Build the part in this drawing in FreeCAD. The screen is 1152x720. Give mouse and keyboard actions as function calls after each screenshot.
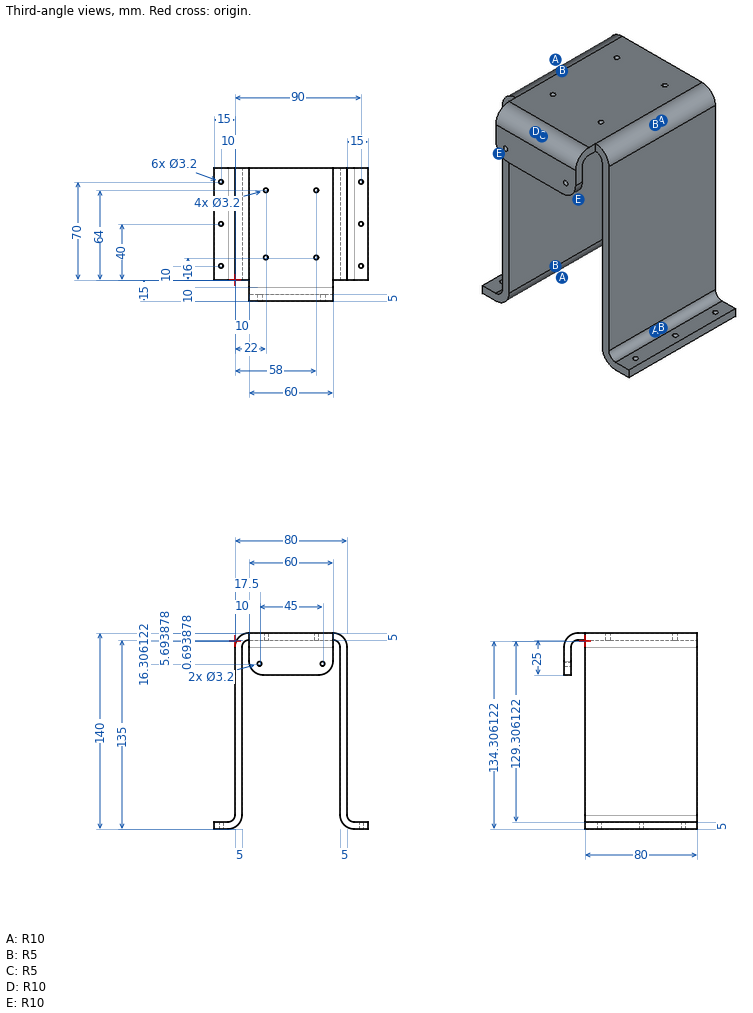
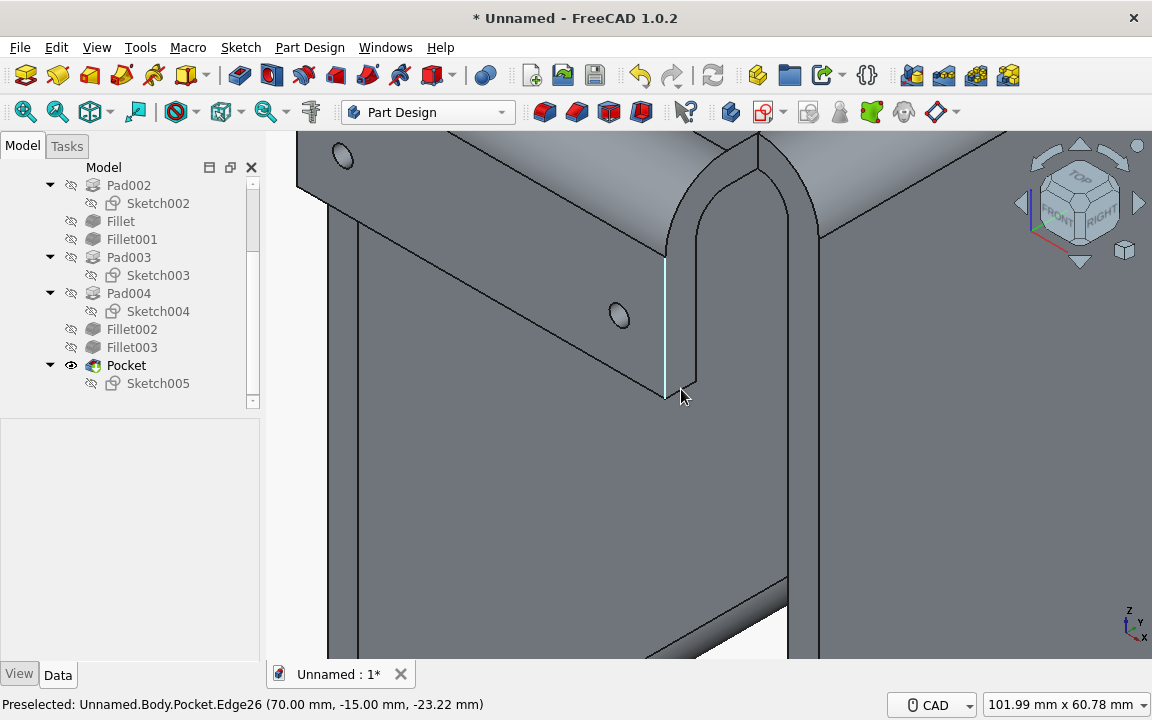
click(26, 112)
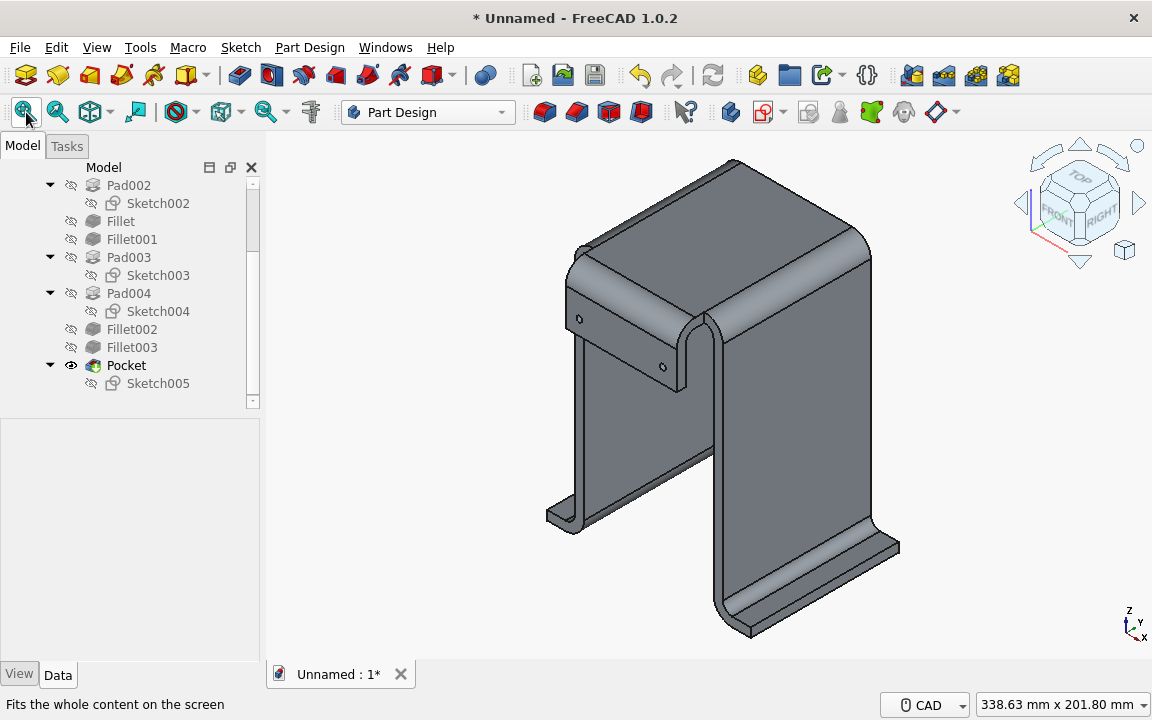
key(2)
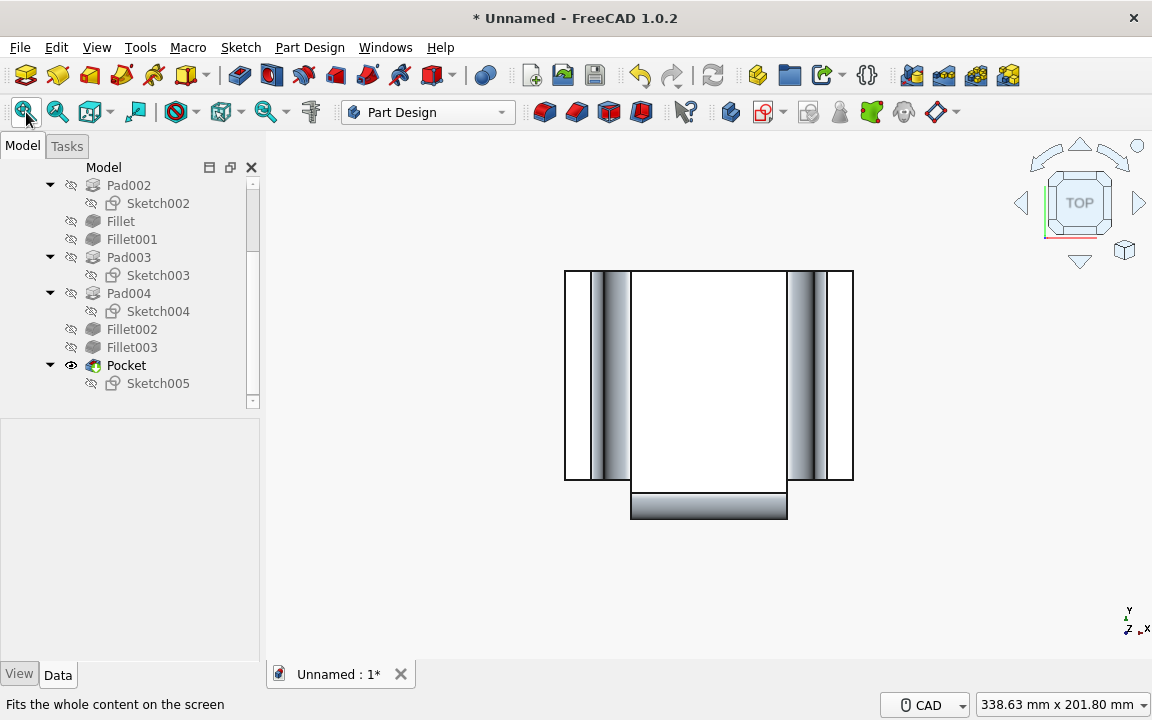
scroll(787, 512, up, 6)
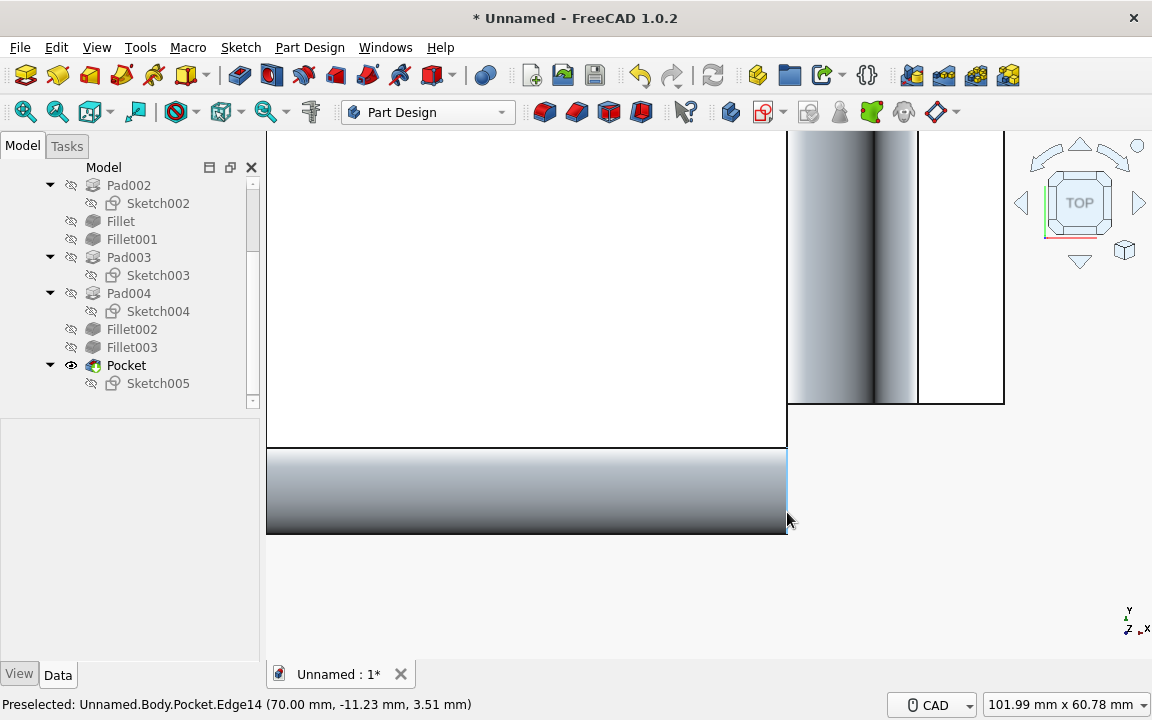
key(v)
key(f)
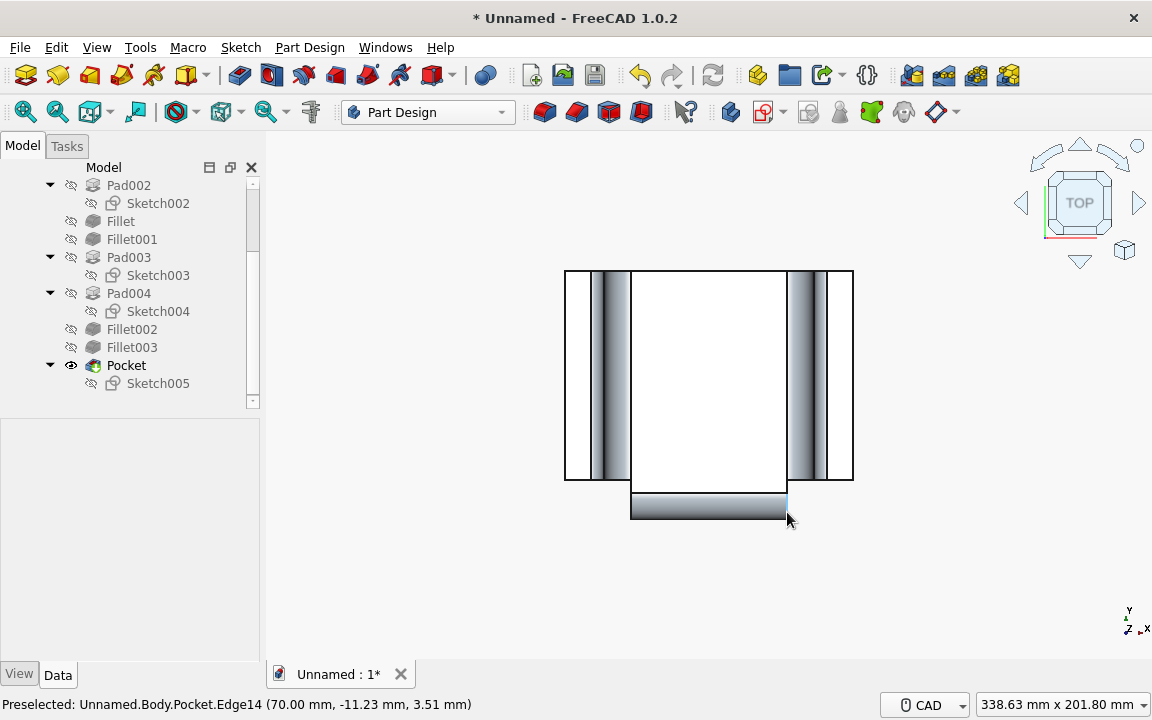
key(0)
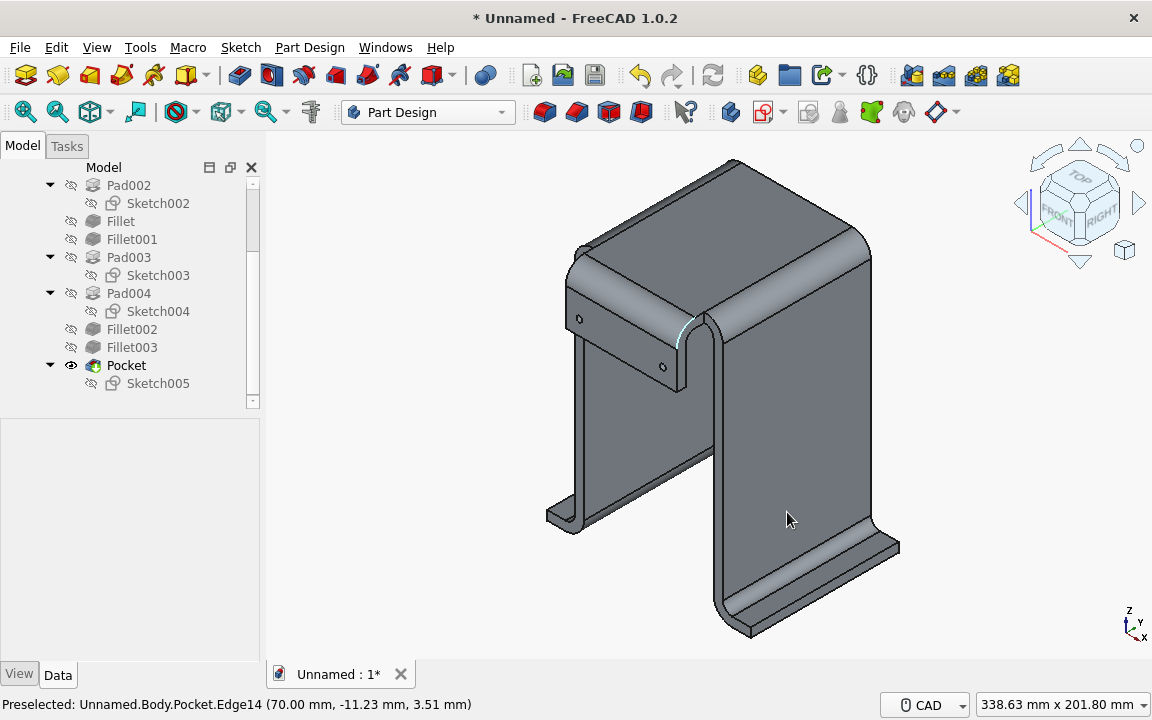
scroll(681, 389, up, 6)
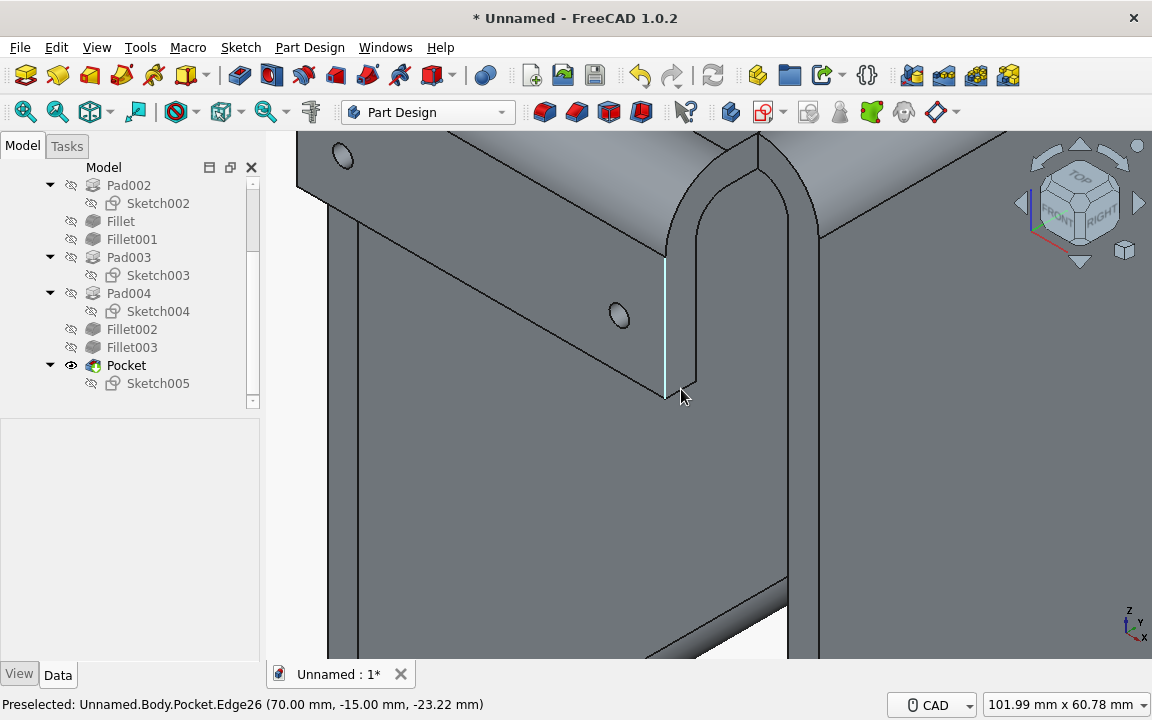
click(26, 112)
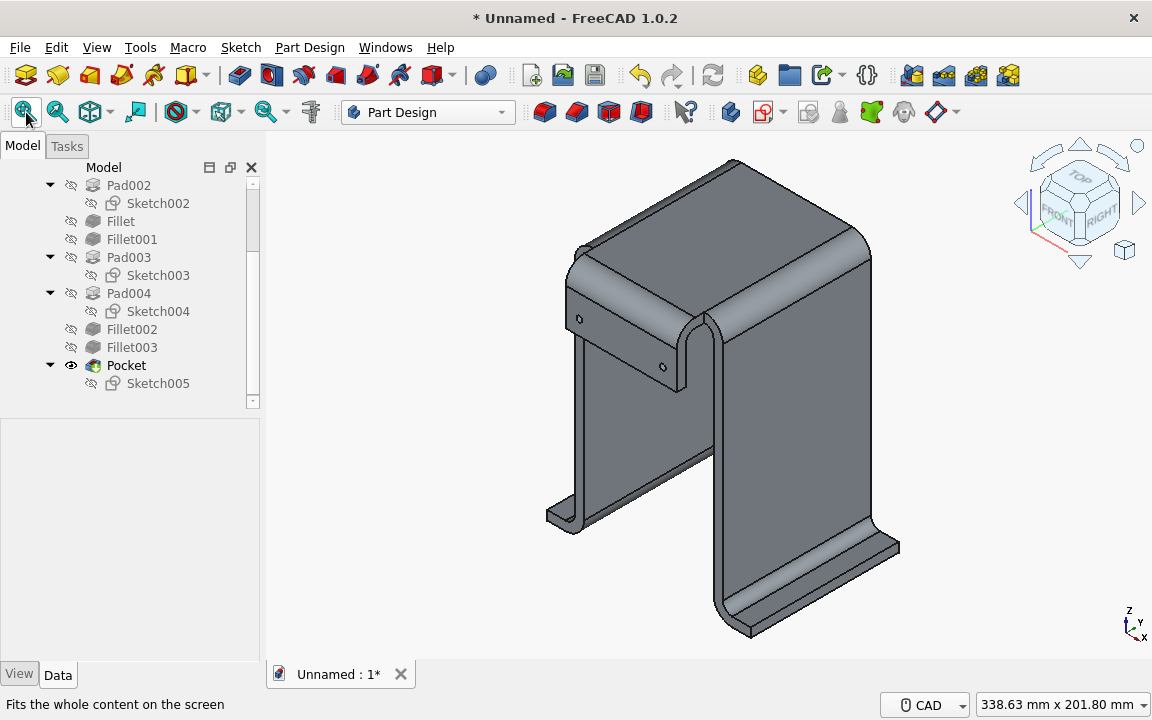
key(1)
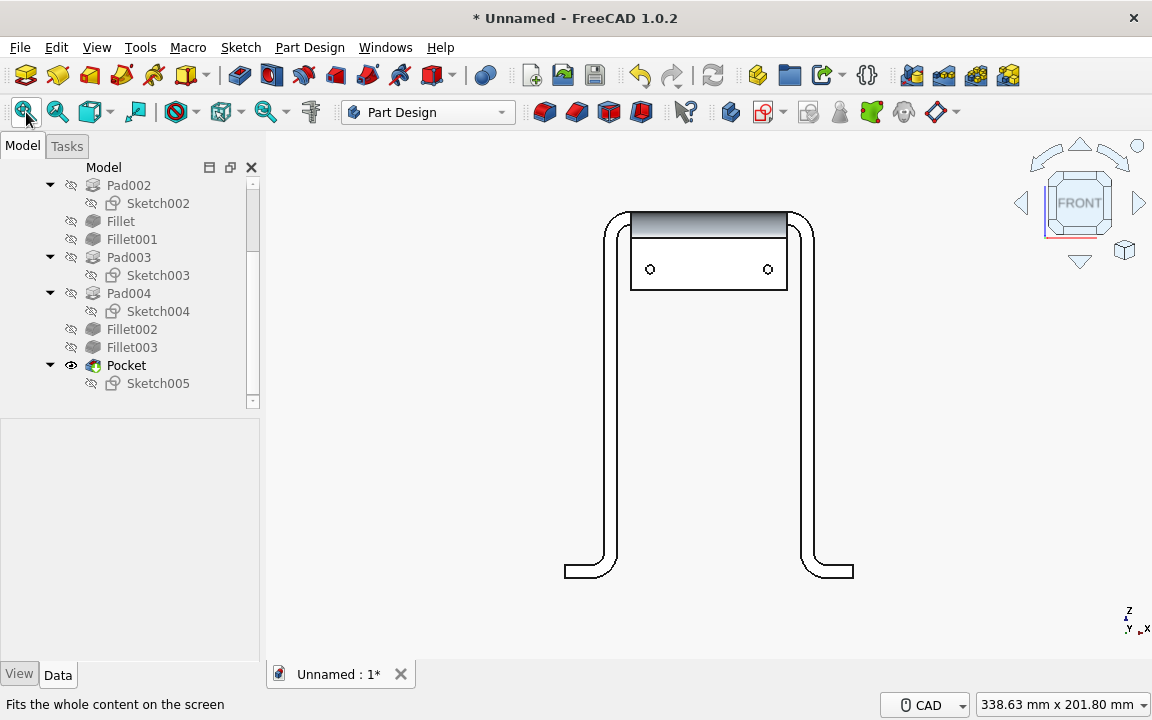
scroll(787, 289, up, 6)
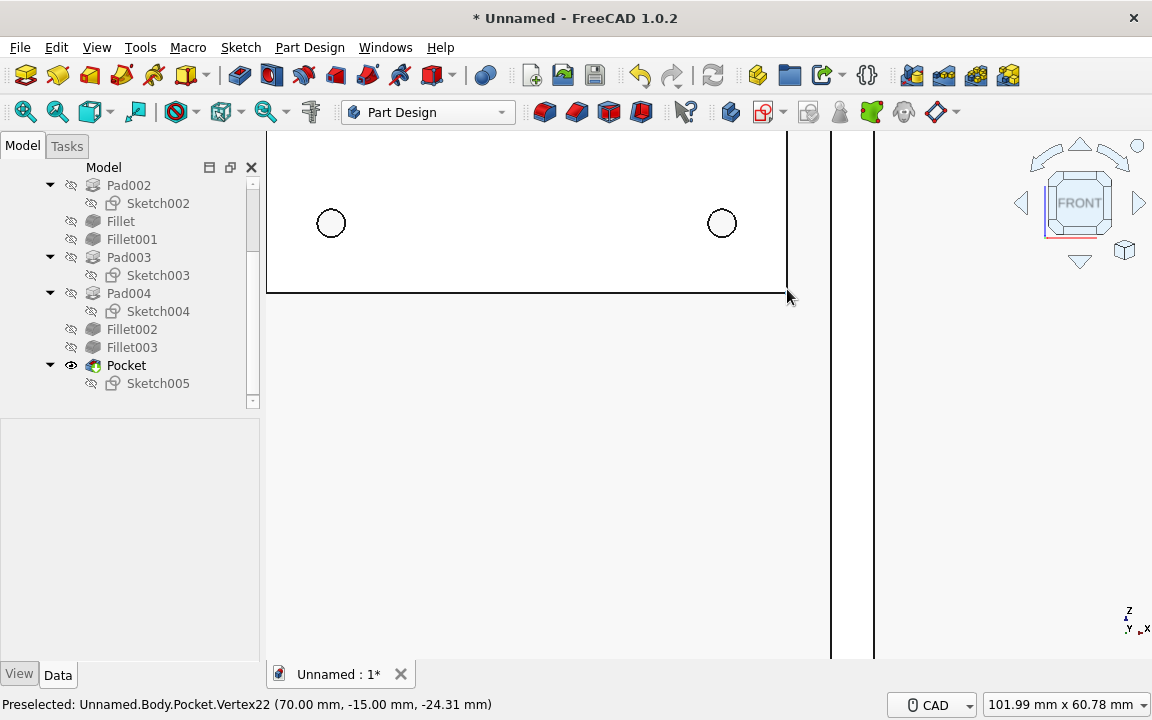
click(26, 112)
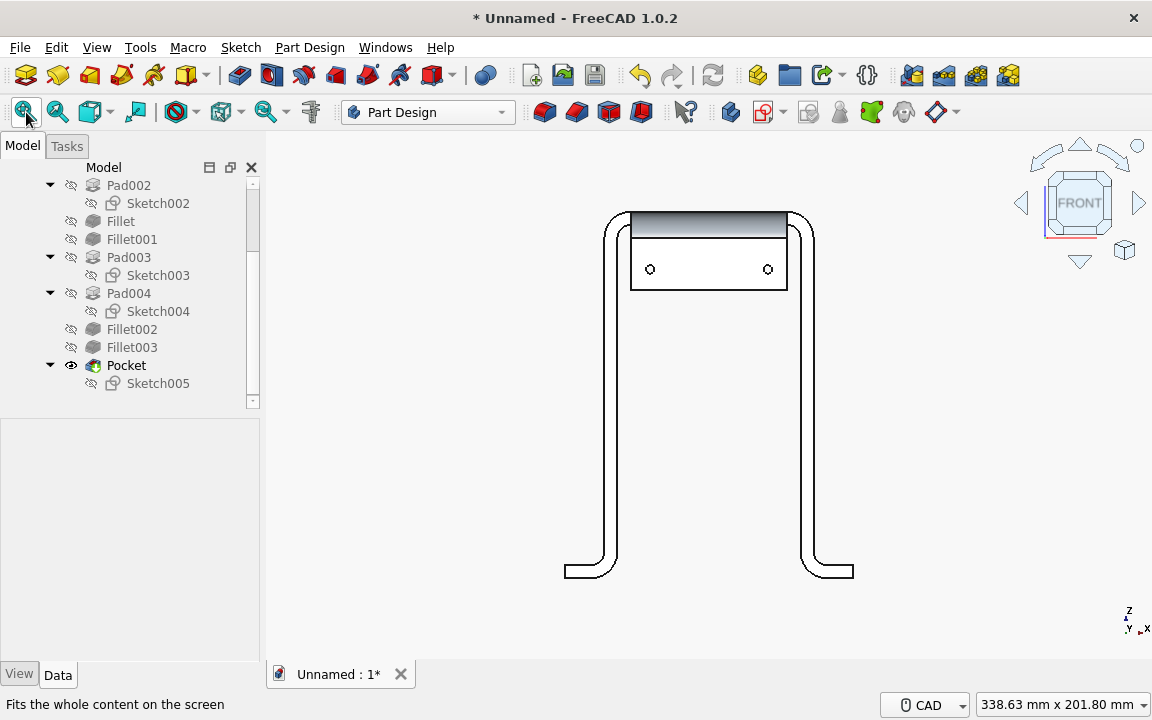
key(3)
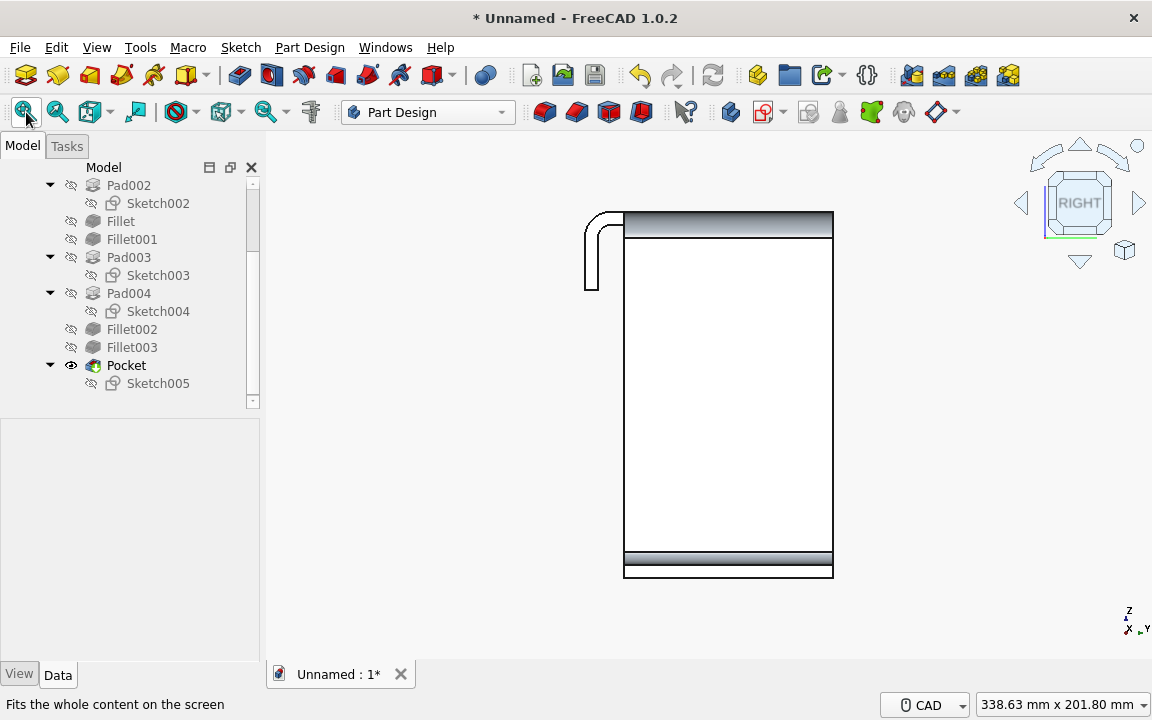
click(591, 289)